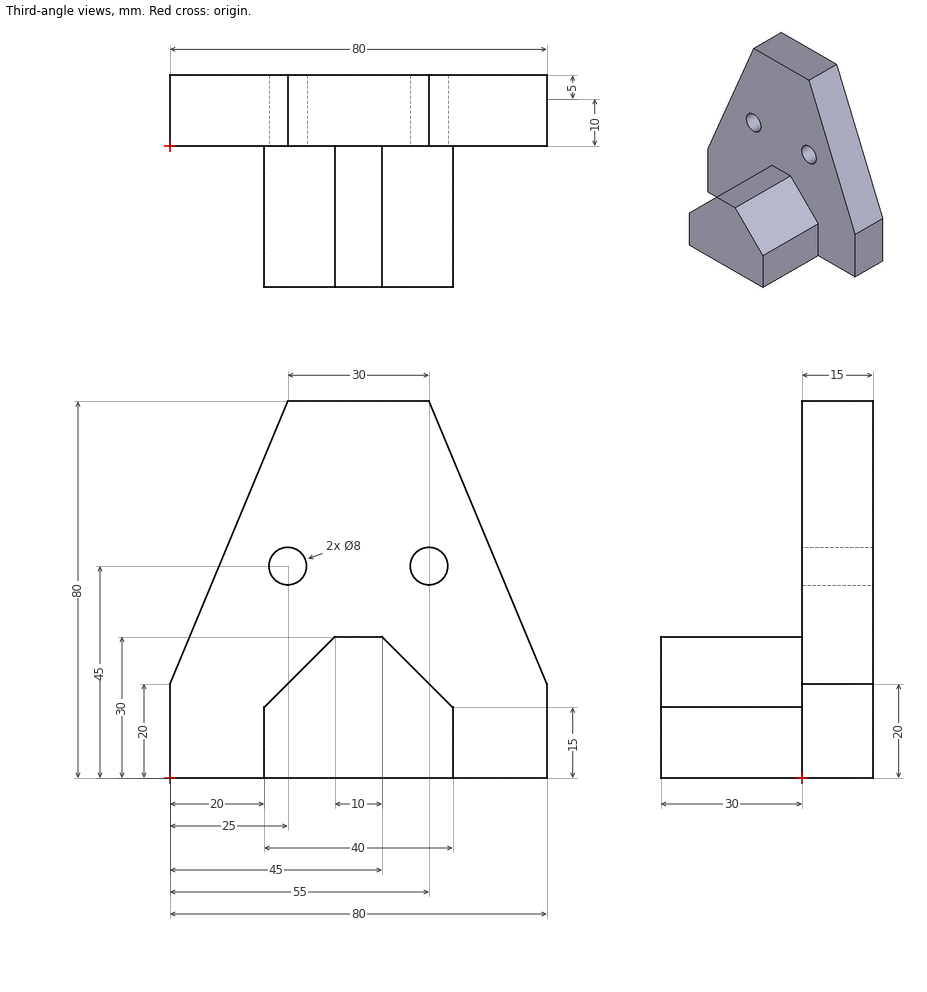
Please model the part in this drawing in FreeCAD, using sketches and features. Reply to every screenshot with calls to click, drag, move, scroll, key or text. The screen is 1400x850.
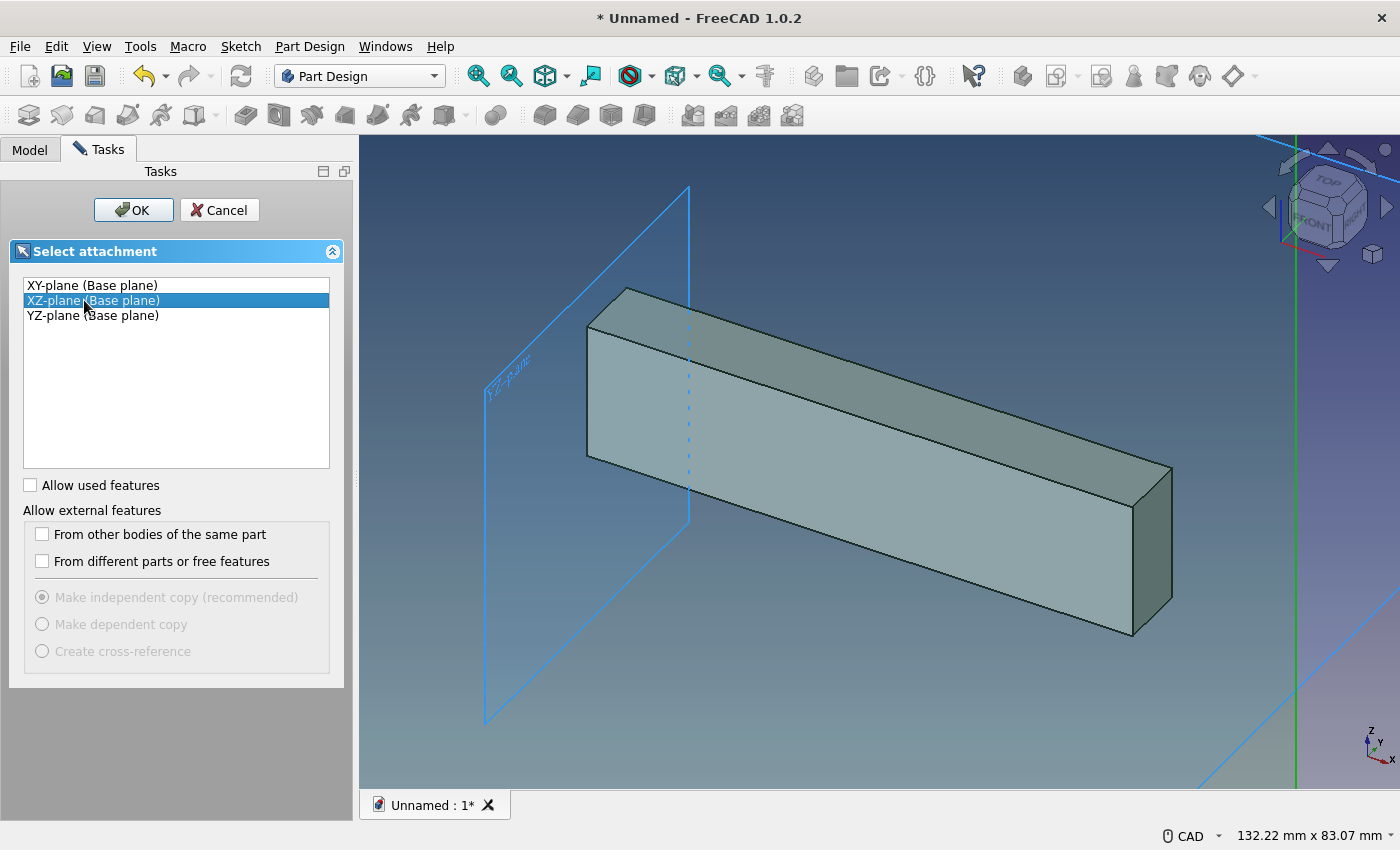
click(134, 210)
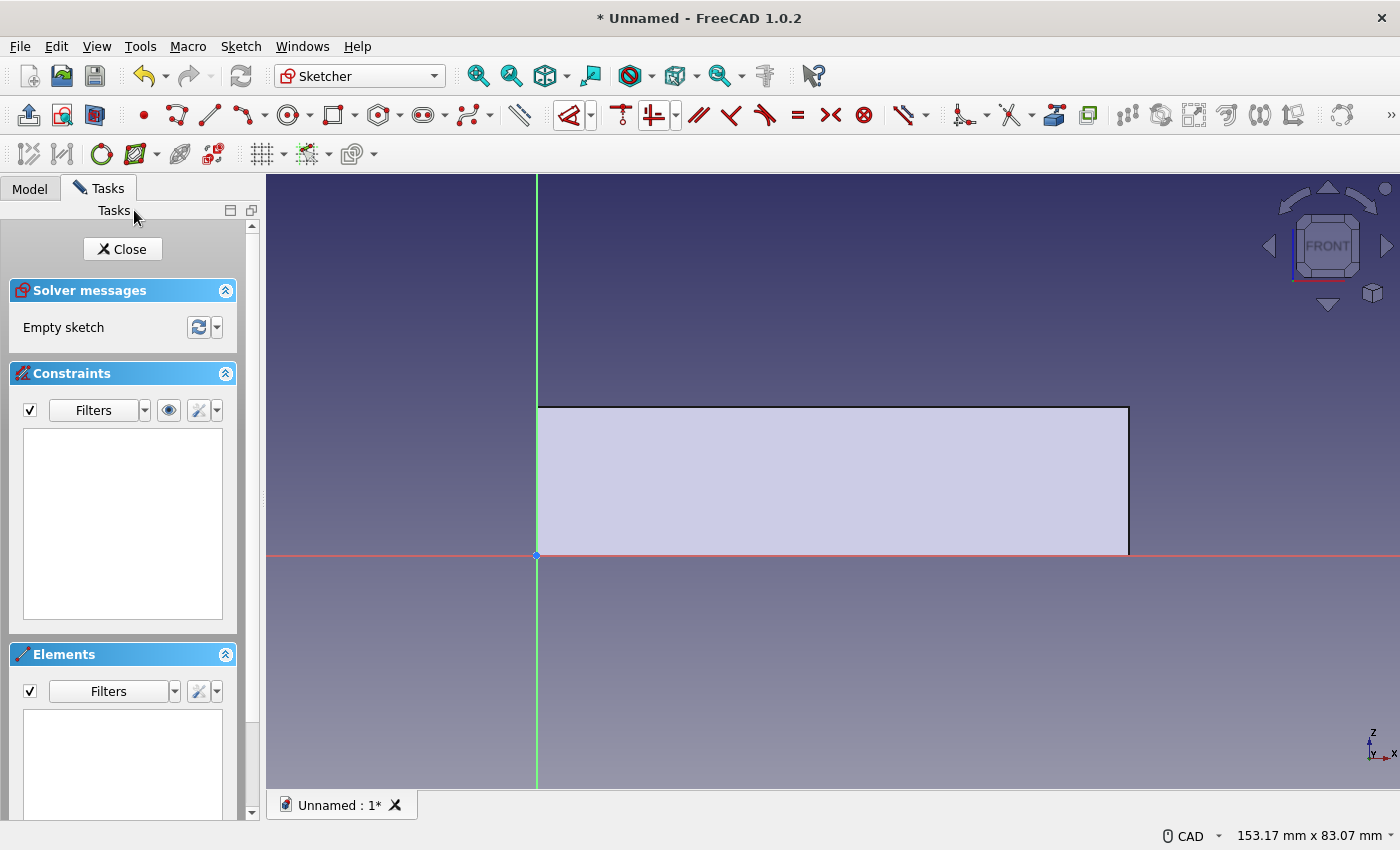
scroll(681, 752, down, 3)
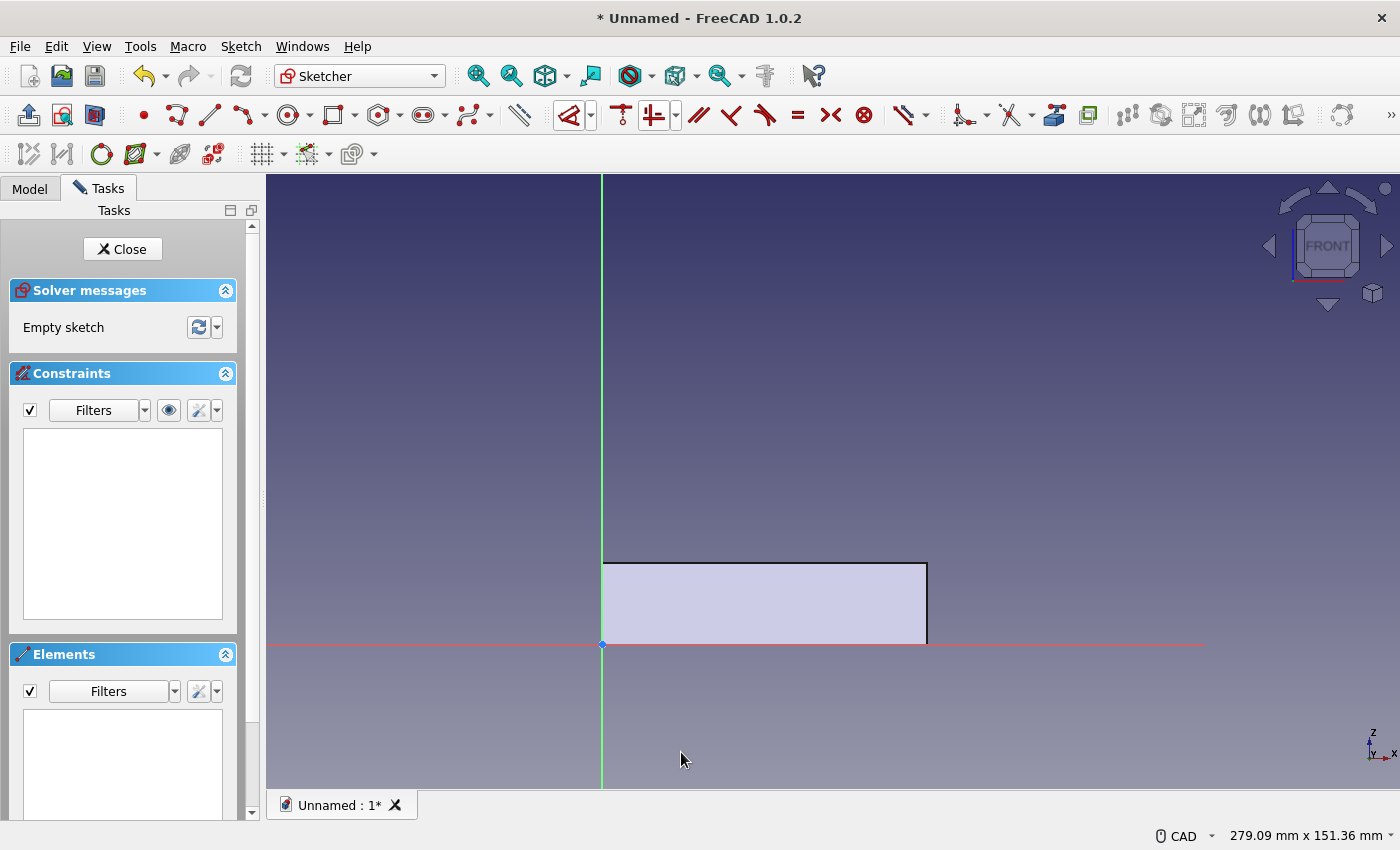
click(177, 116)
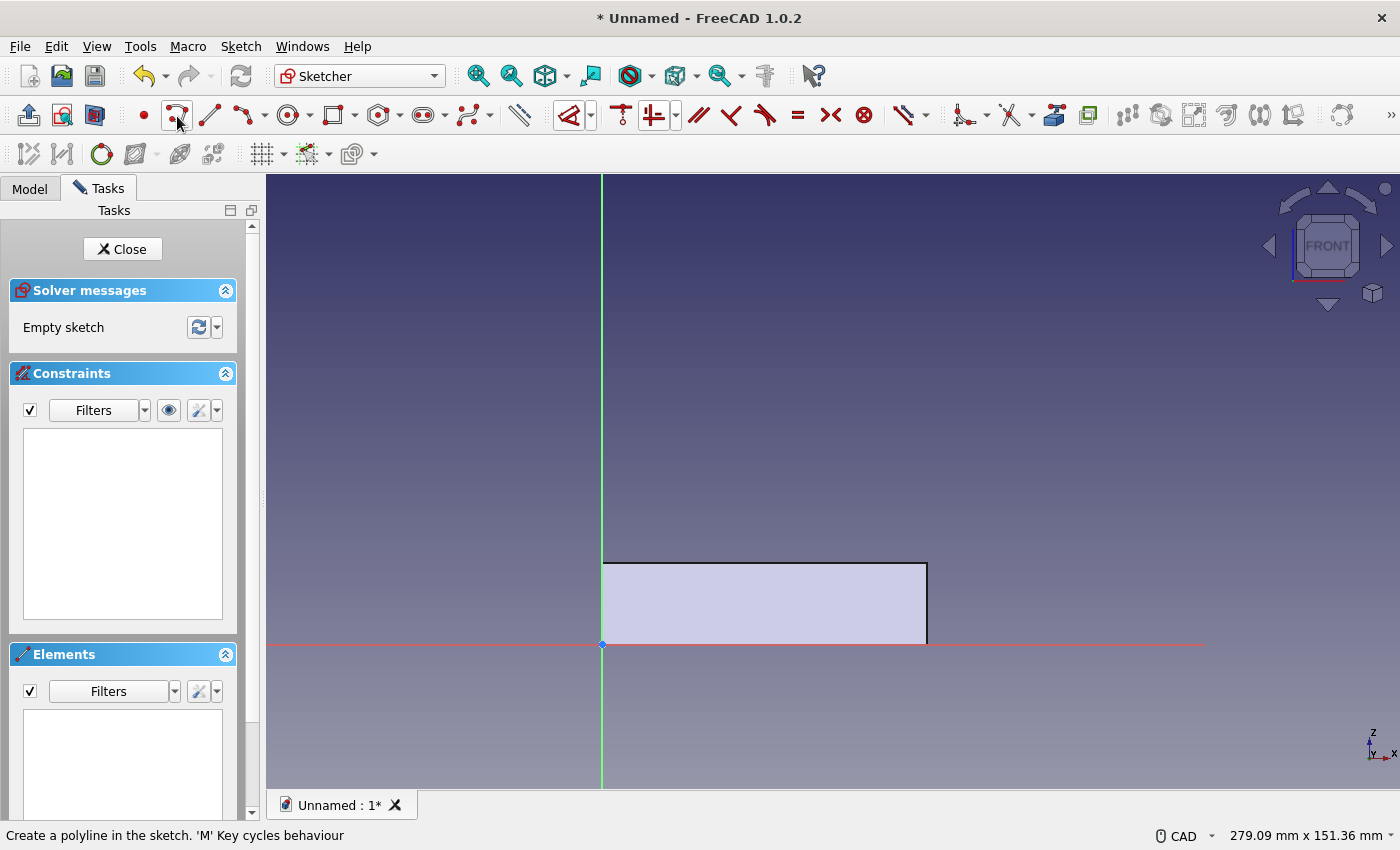
click(602, 563)
click(927, 563)
click(826, 320)
click(704, 320)
click(602, 564)
key(Escape)
key(Escape)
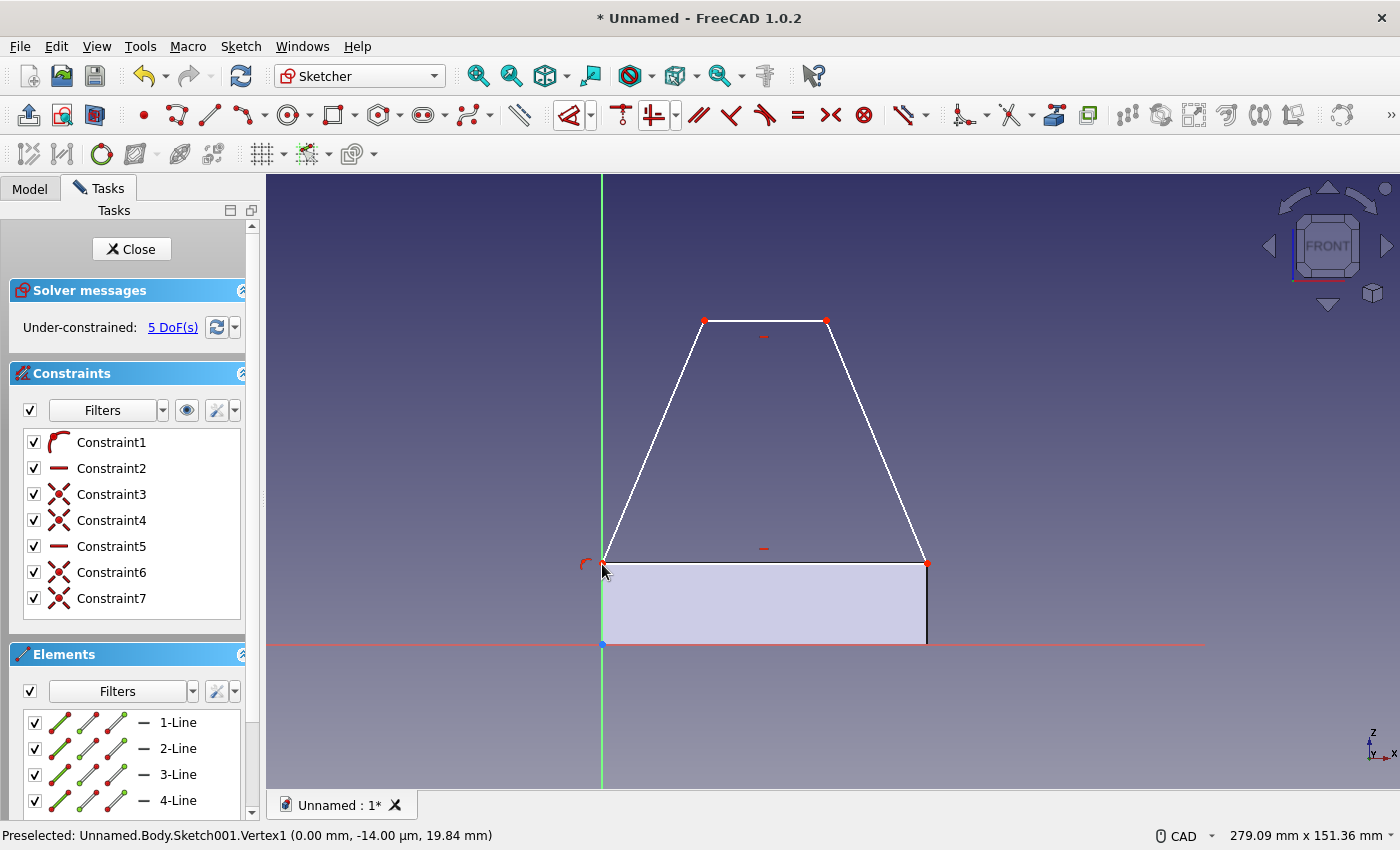
click(700, 564)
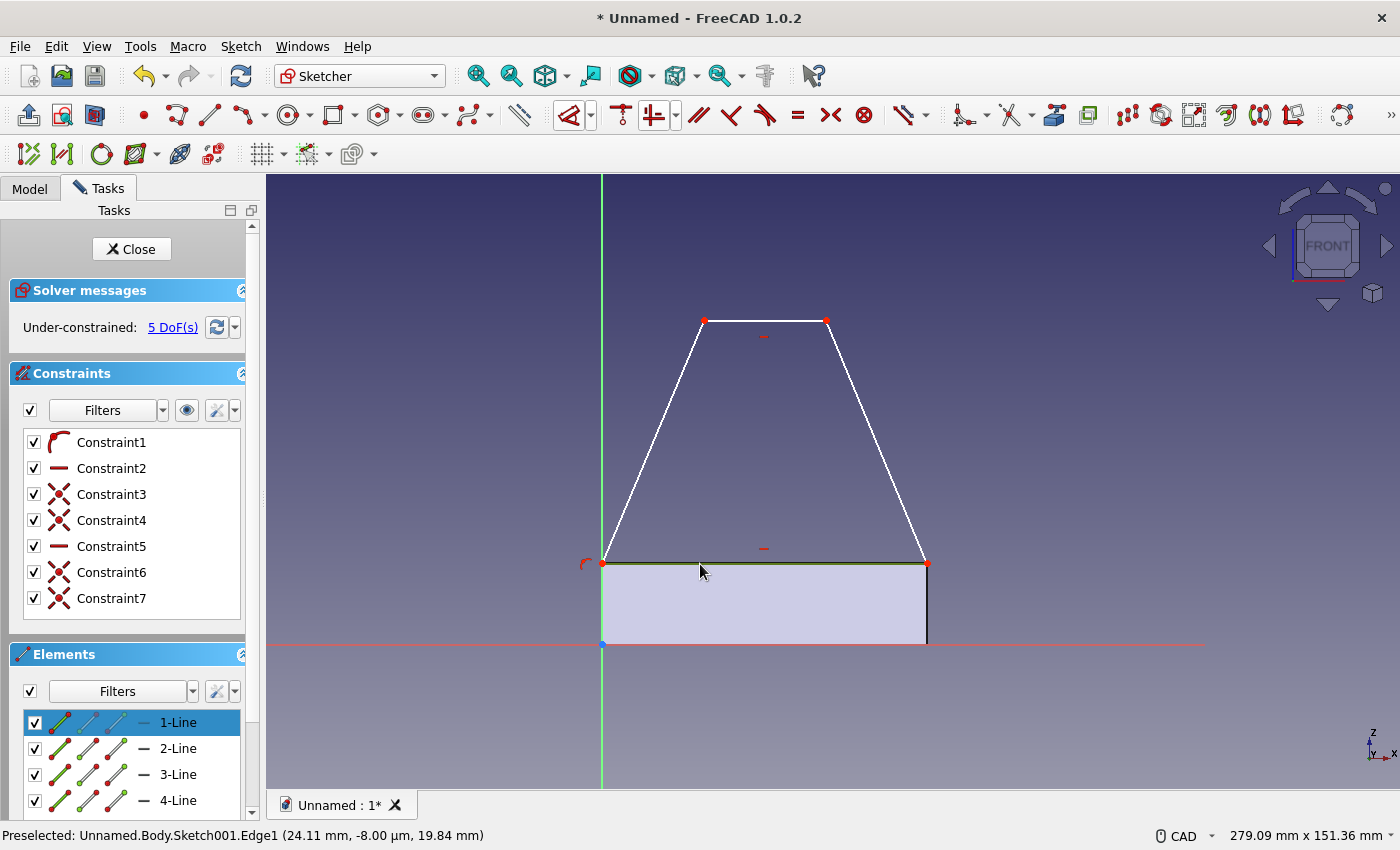
click(590, 116)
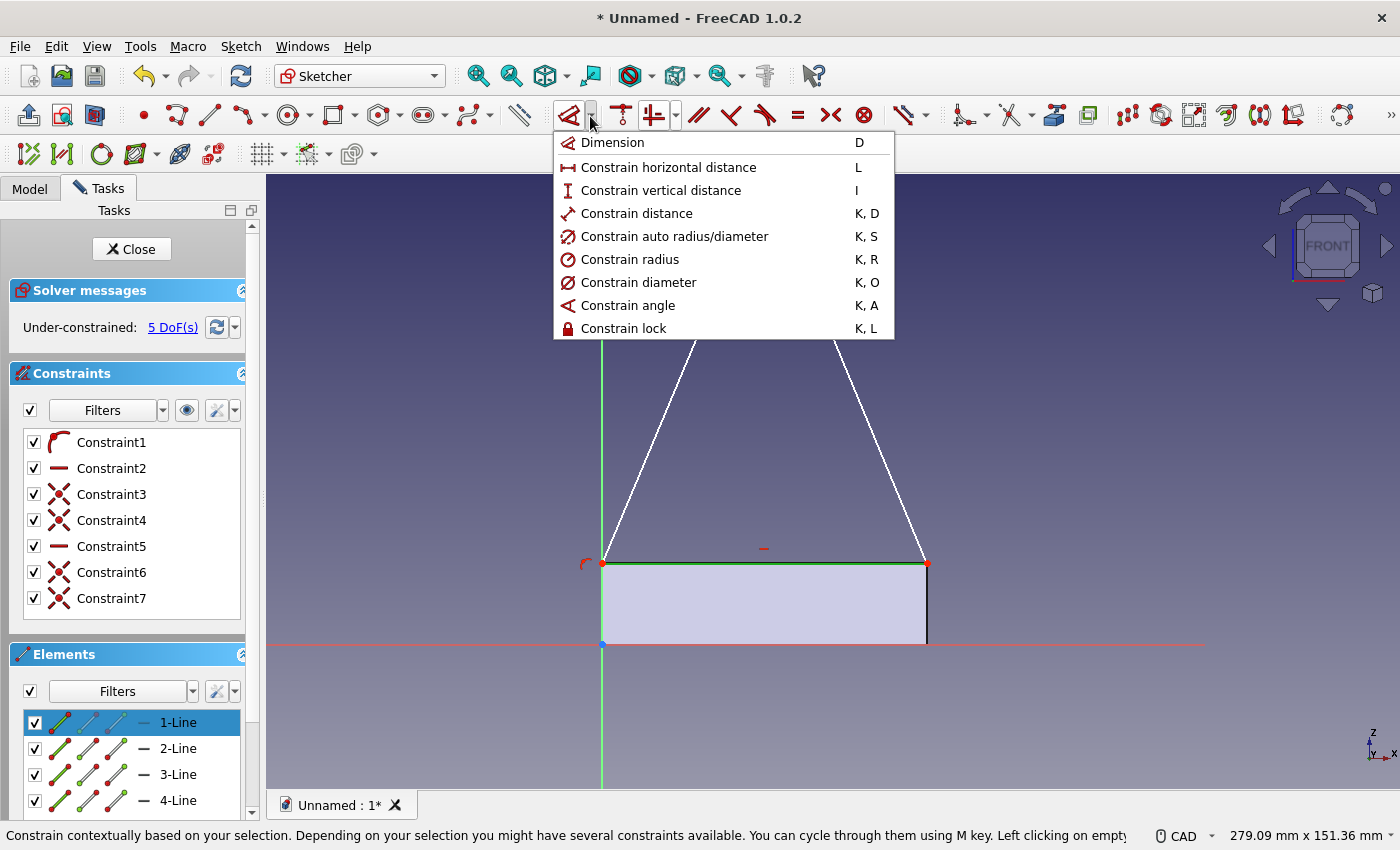
click(724, 168)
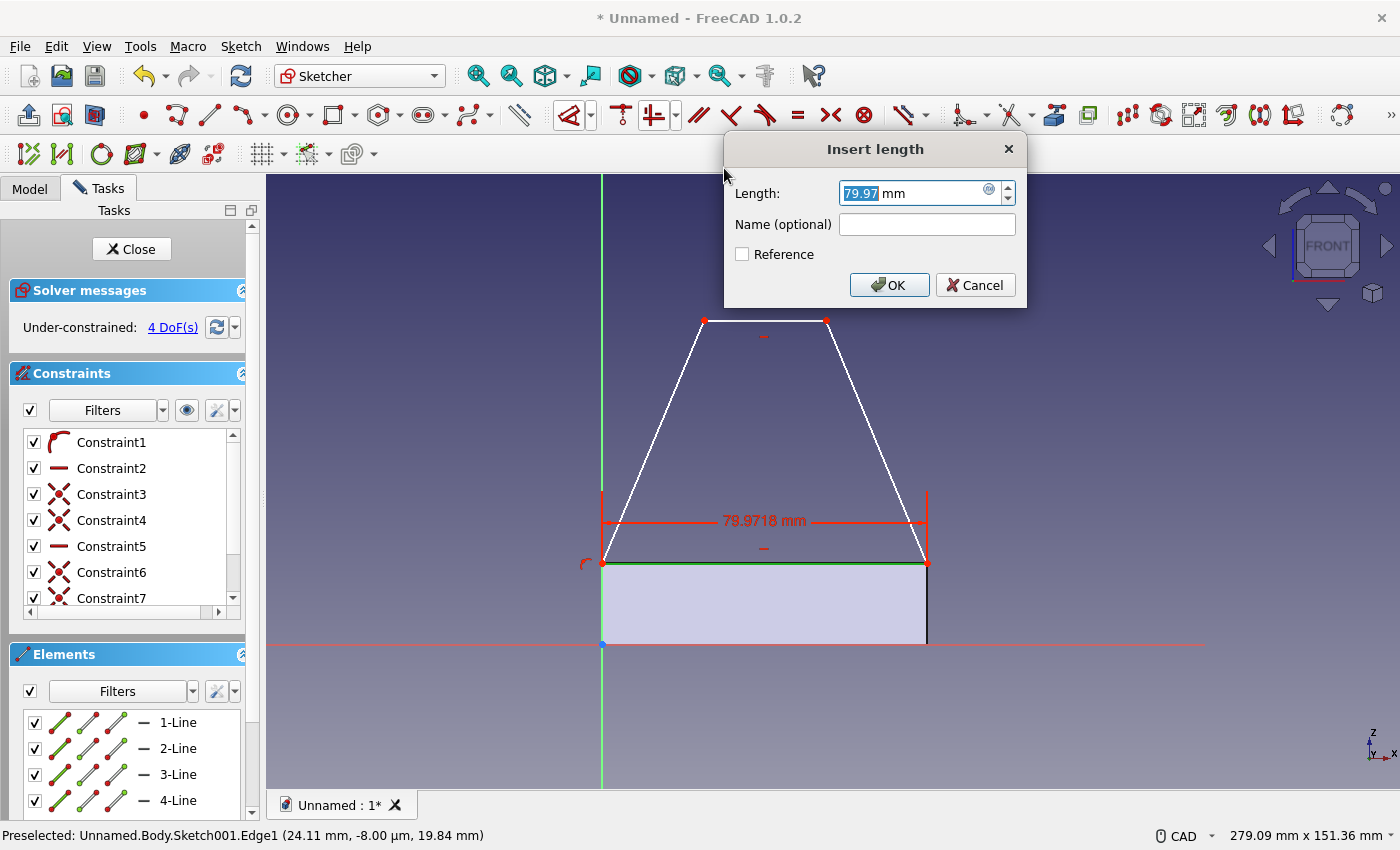
text(80)
key(Return)